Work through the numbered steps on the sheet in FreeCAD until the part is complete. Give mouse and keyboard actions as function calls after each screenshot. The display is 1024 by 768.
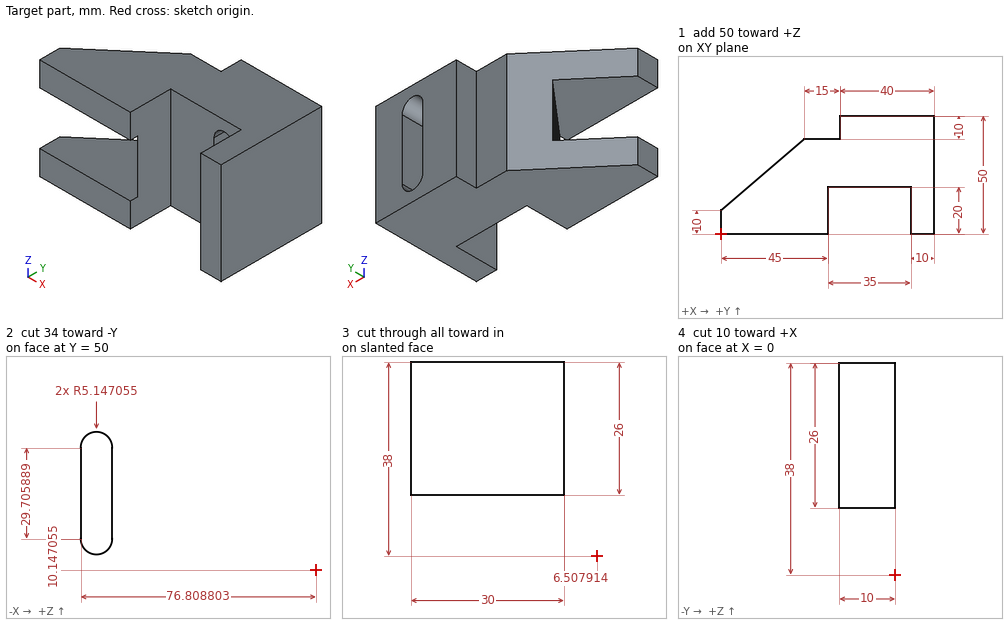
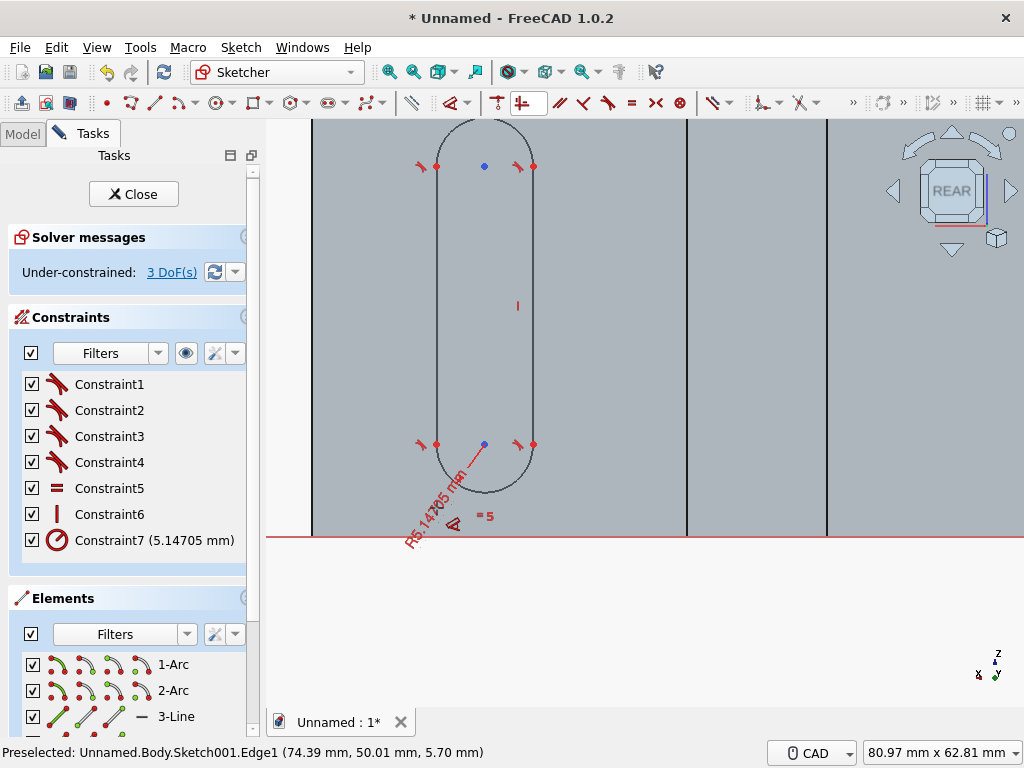
click(437, 361)
click(403, 305)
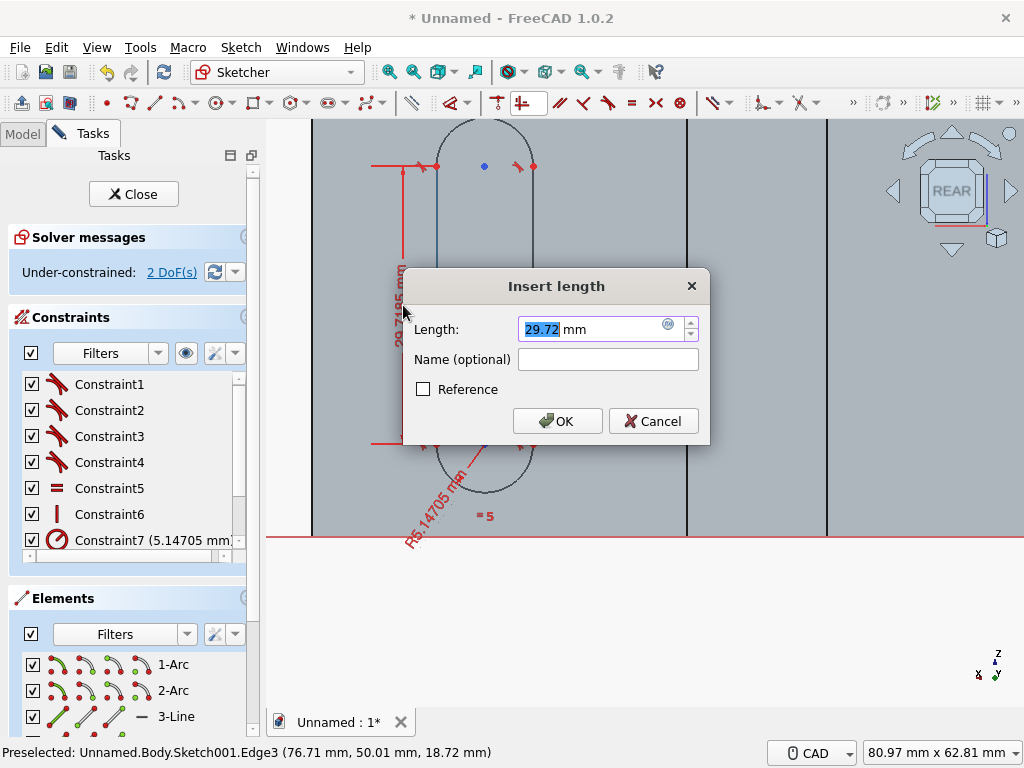
text(29.705889)
key(Return)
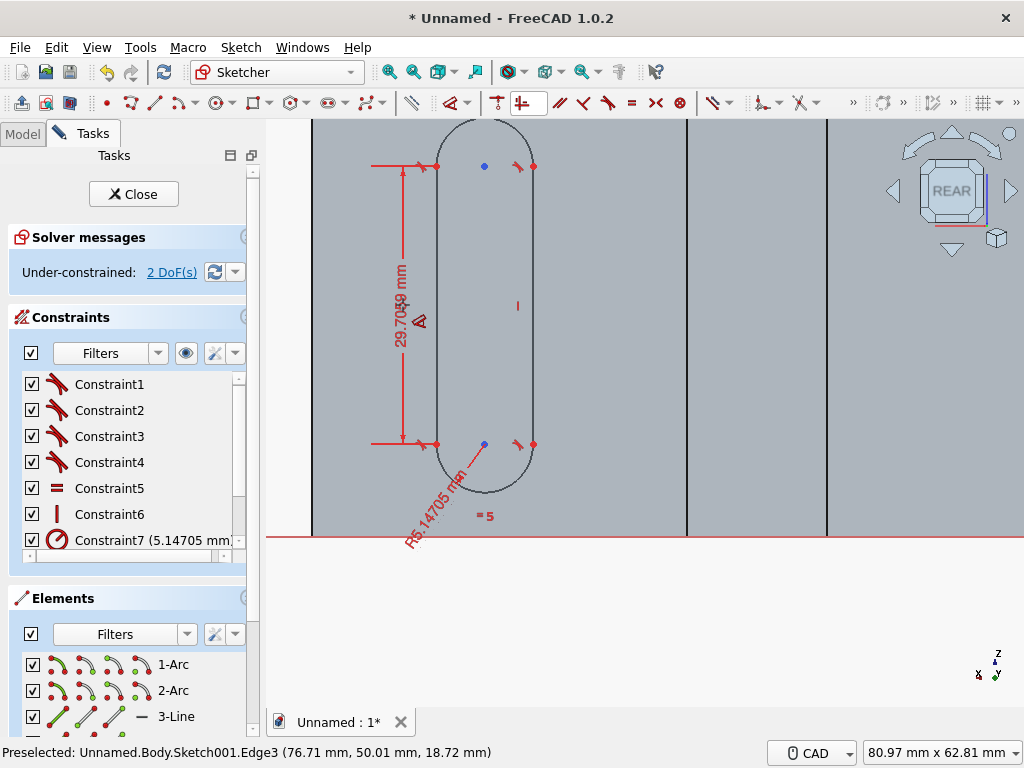
click(437, 444)
click(648, 571)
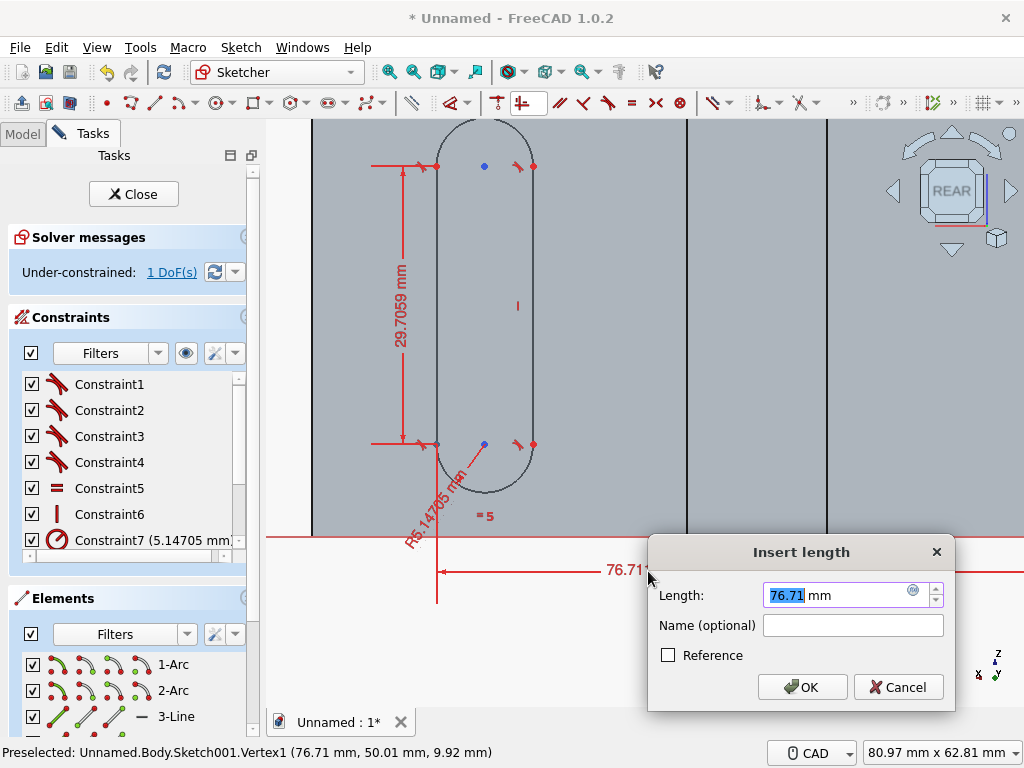
text(76.808803)
key(Return)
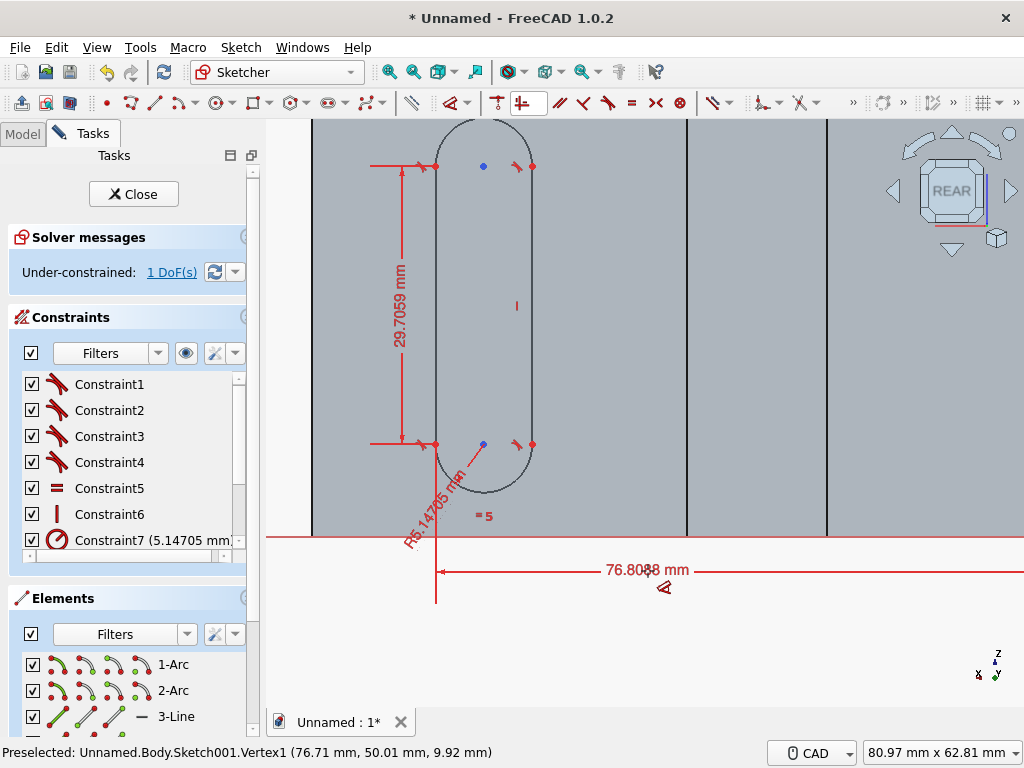
click(436, 444)
click(402, 469)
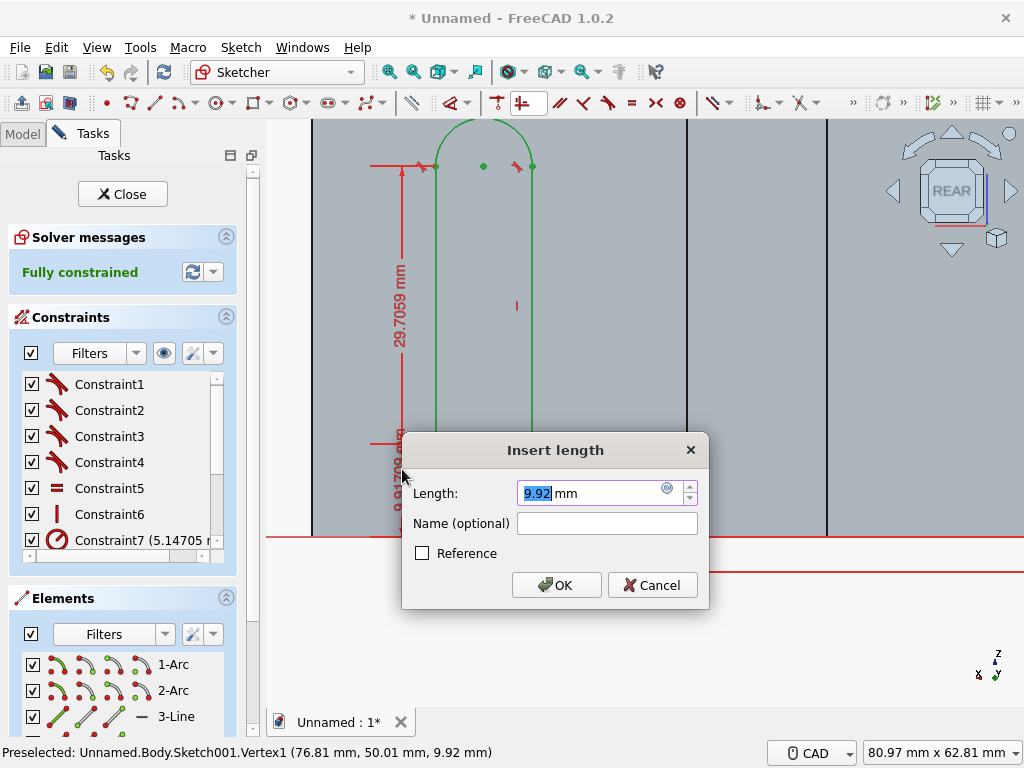
text(10.147055)
key(Return)
key(Escape)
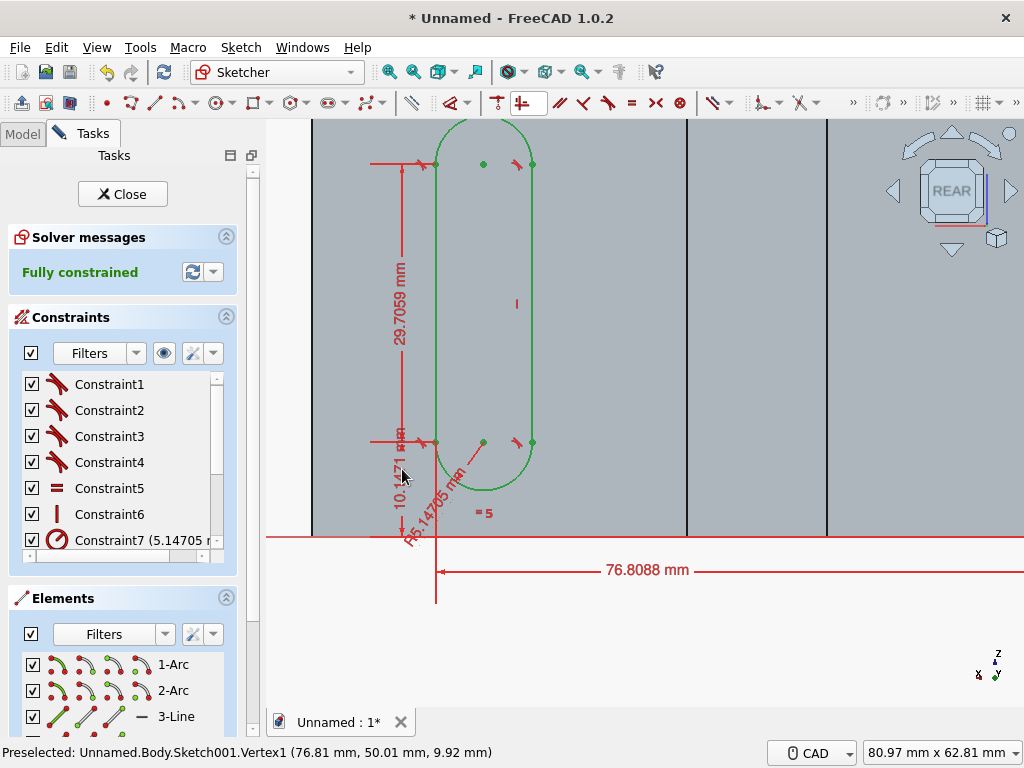
click(123, 194)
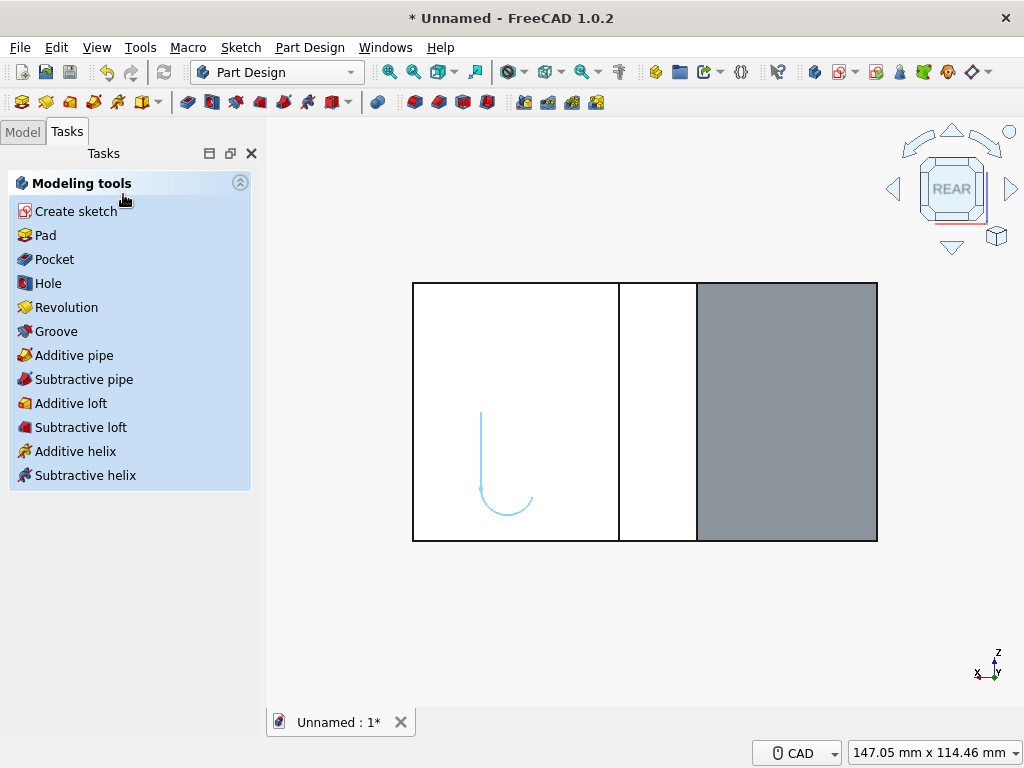
click(188, 102)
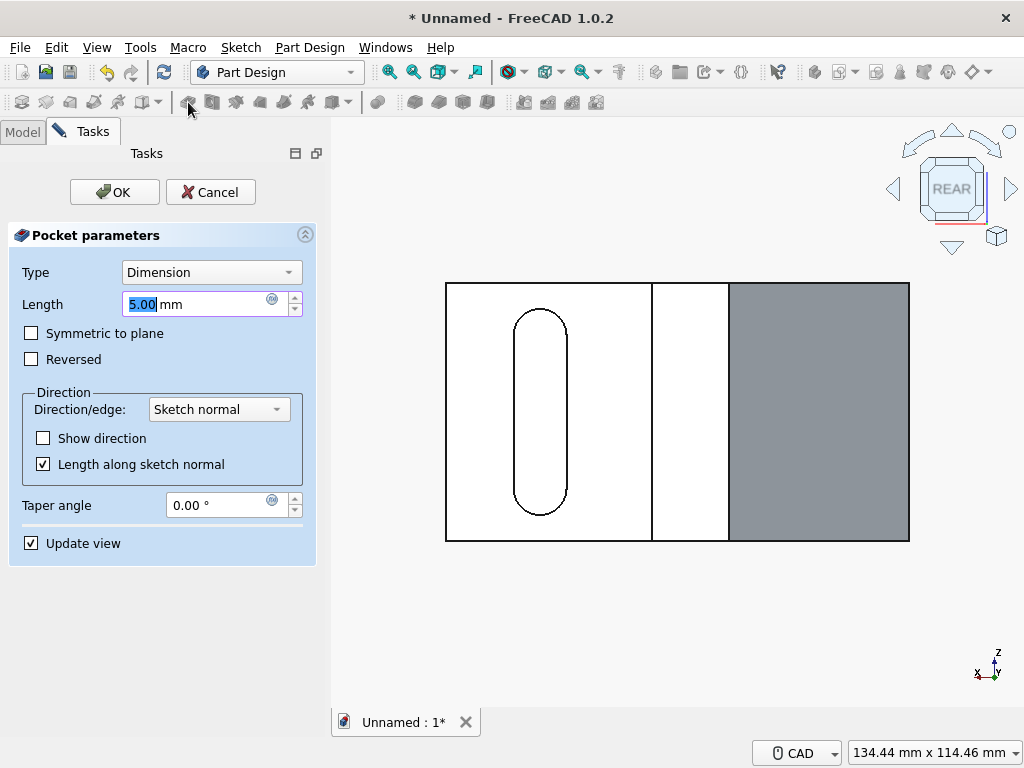
text(34)
key(Tab)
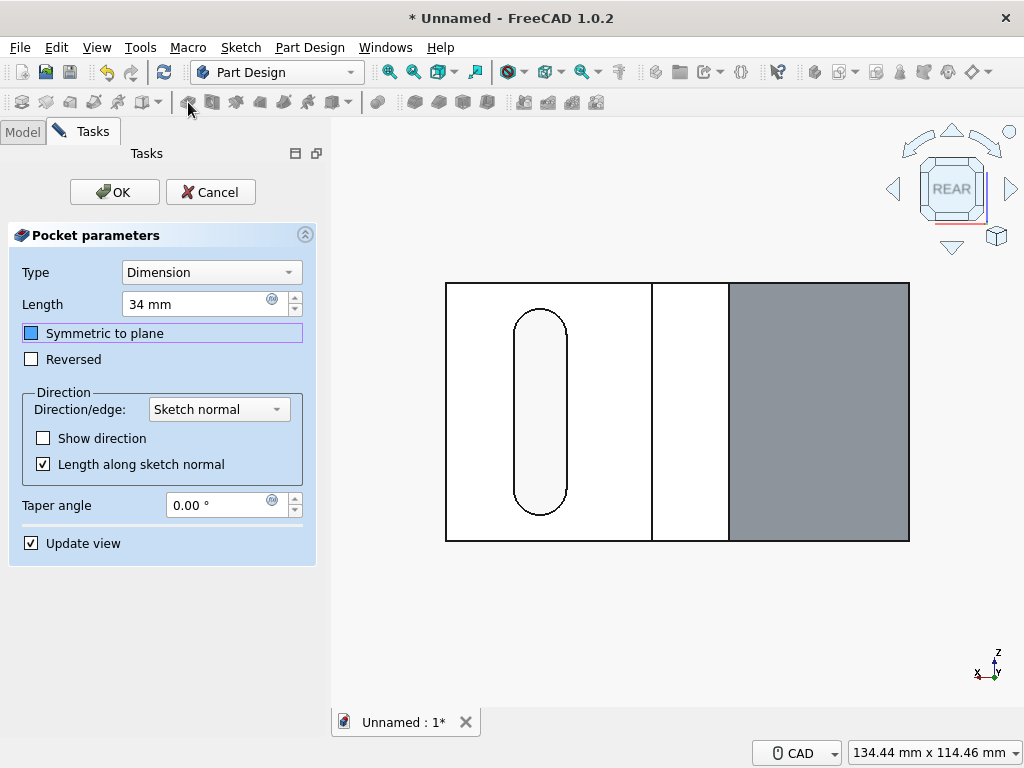
click(115, 192)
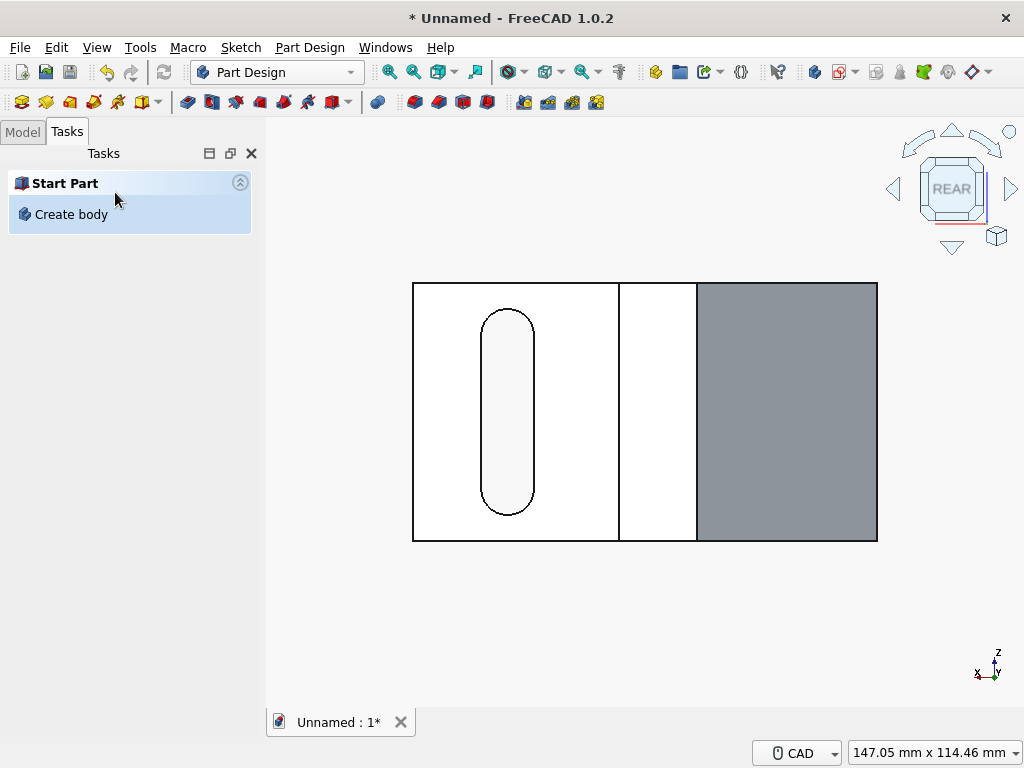
click(787, 411)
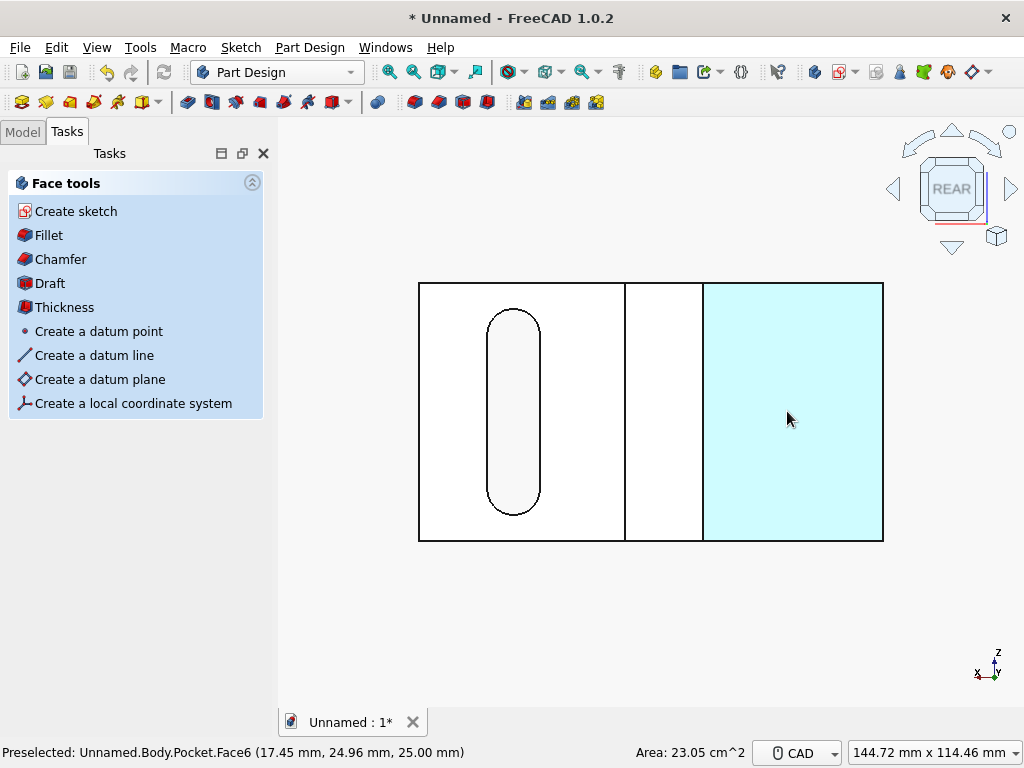
click(840, 72)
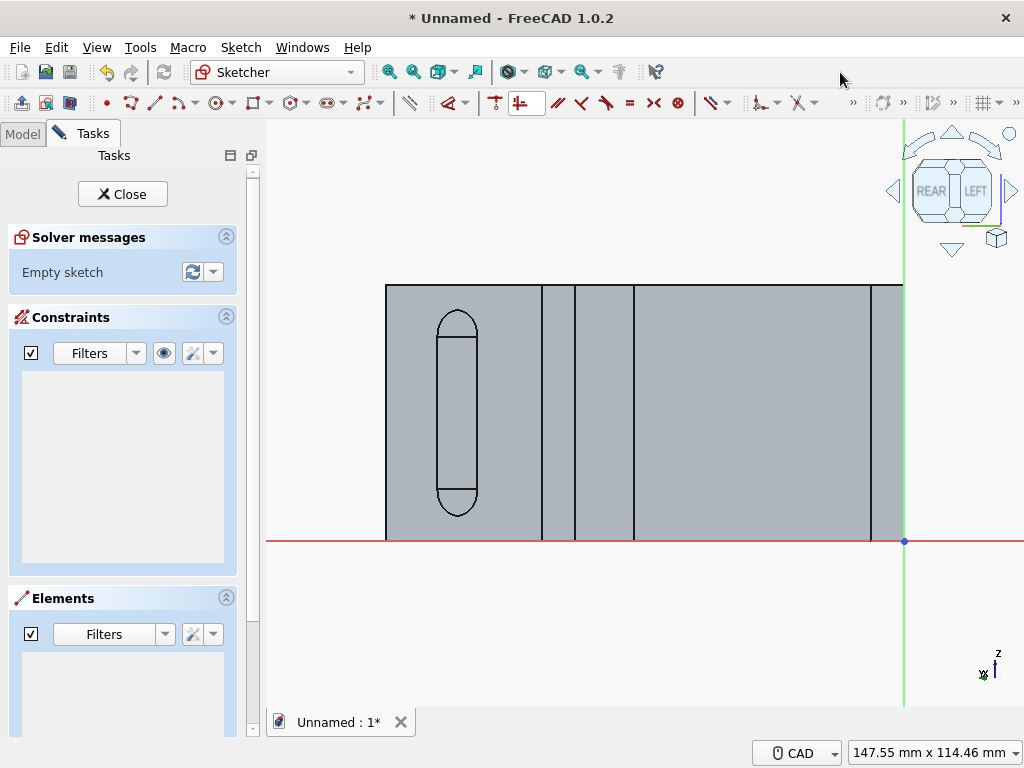
click(70, 104)